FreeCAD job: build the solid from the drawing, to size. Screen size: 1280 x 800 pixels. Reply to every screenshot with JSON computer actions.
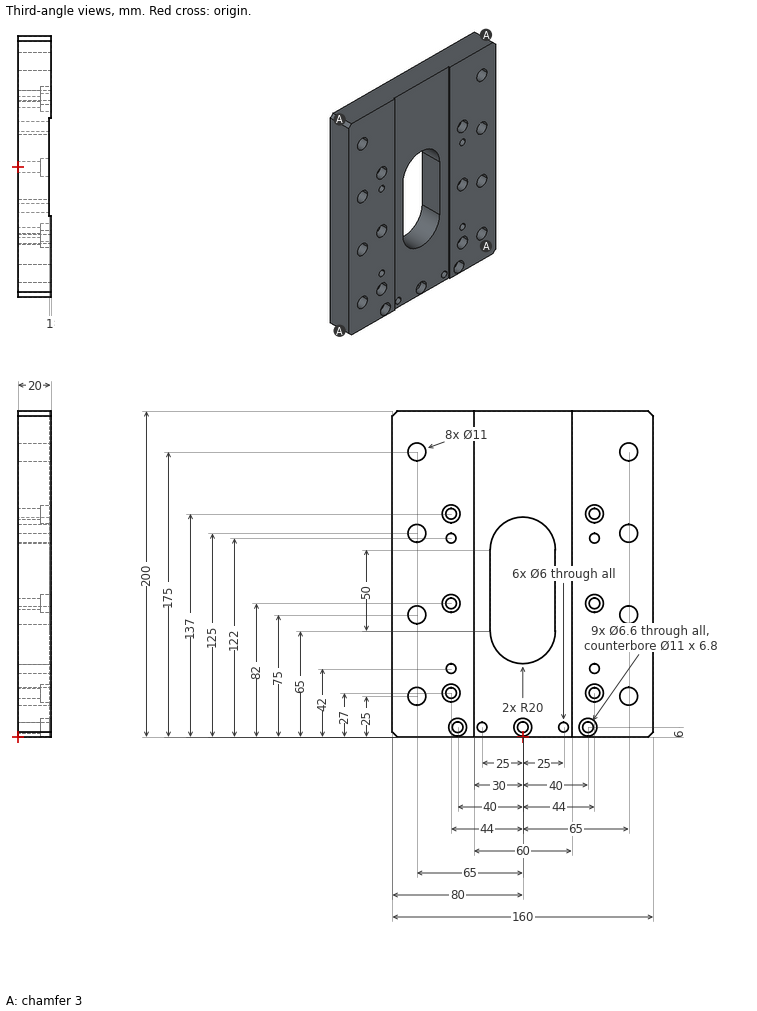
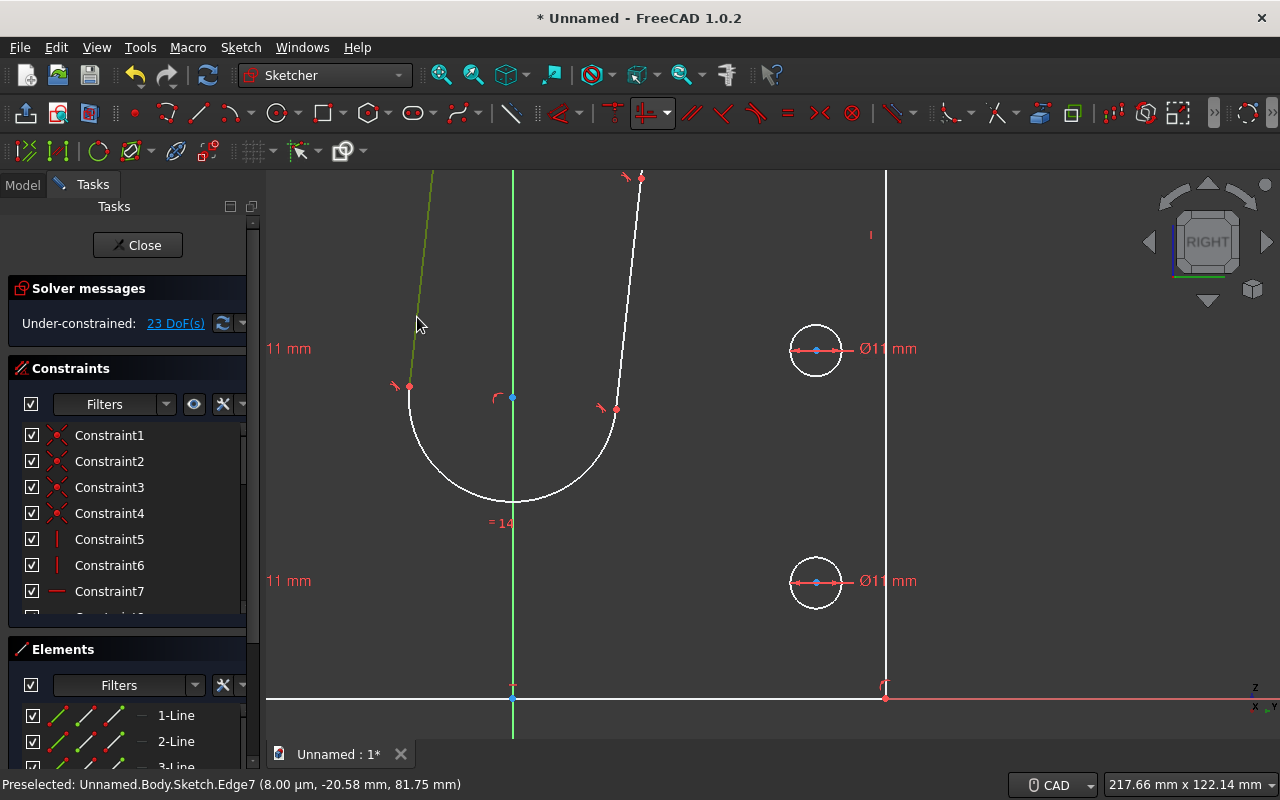
{"action": "left_click", "coordinate": [670, 114]}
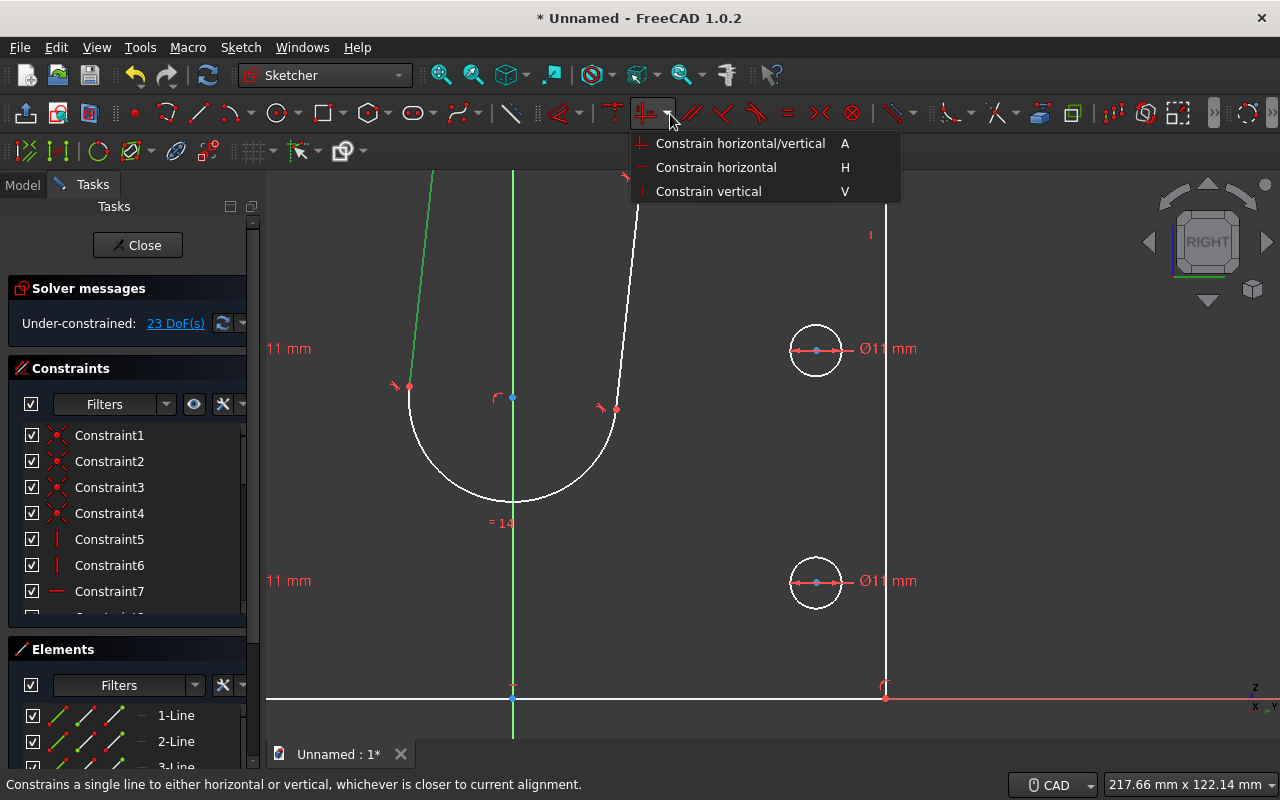
{"action": "left_click", "coordinate": [766, 191]}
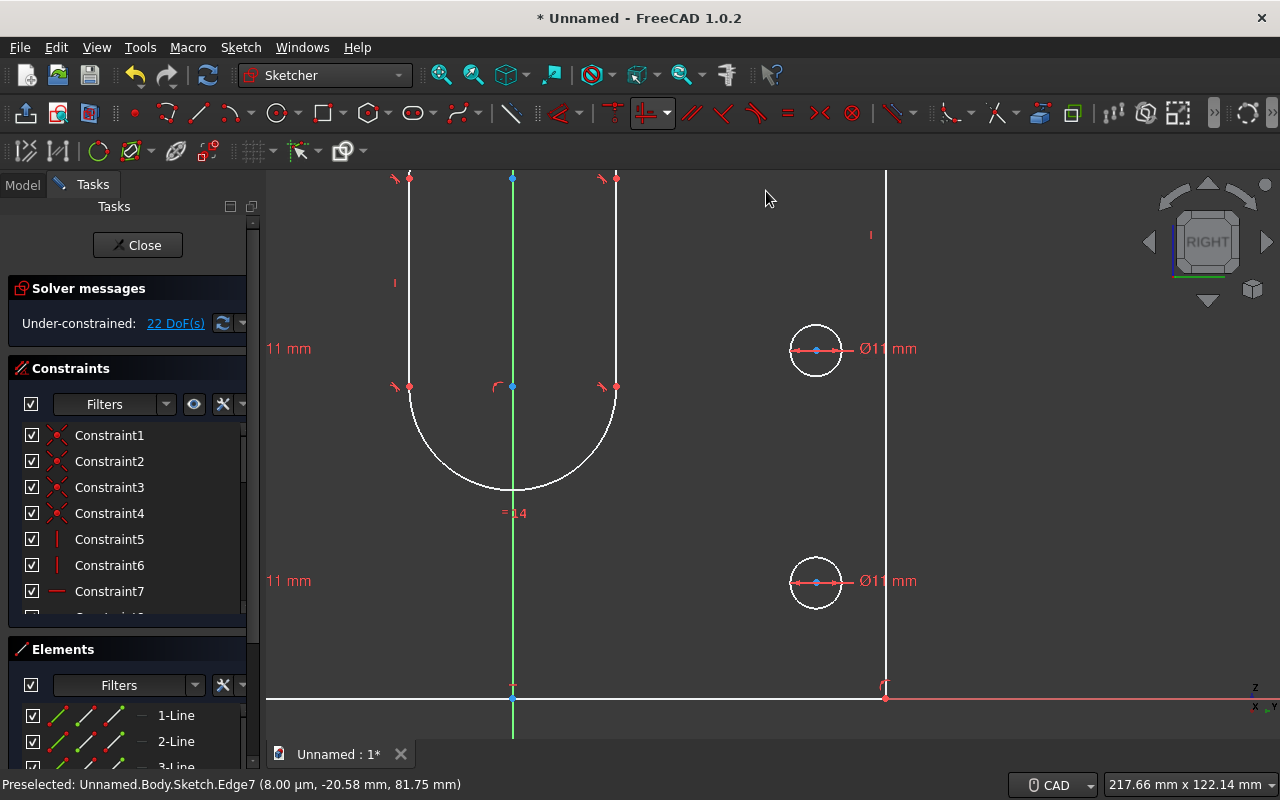
{"action": "scroll", "coordinate": [816, 583], "scroll_direction": "down", "scroll_amount": 5}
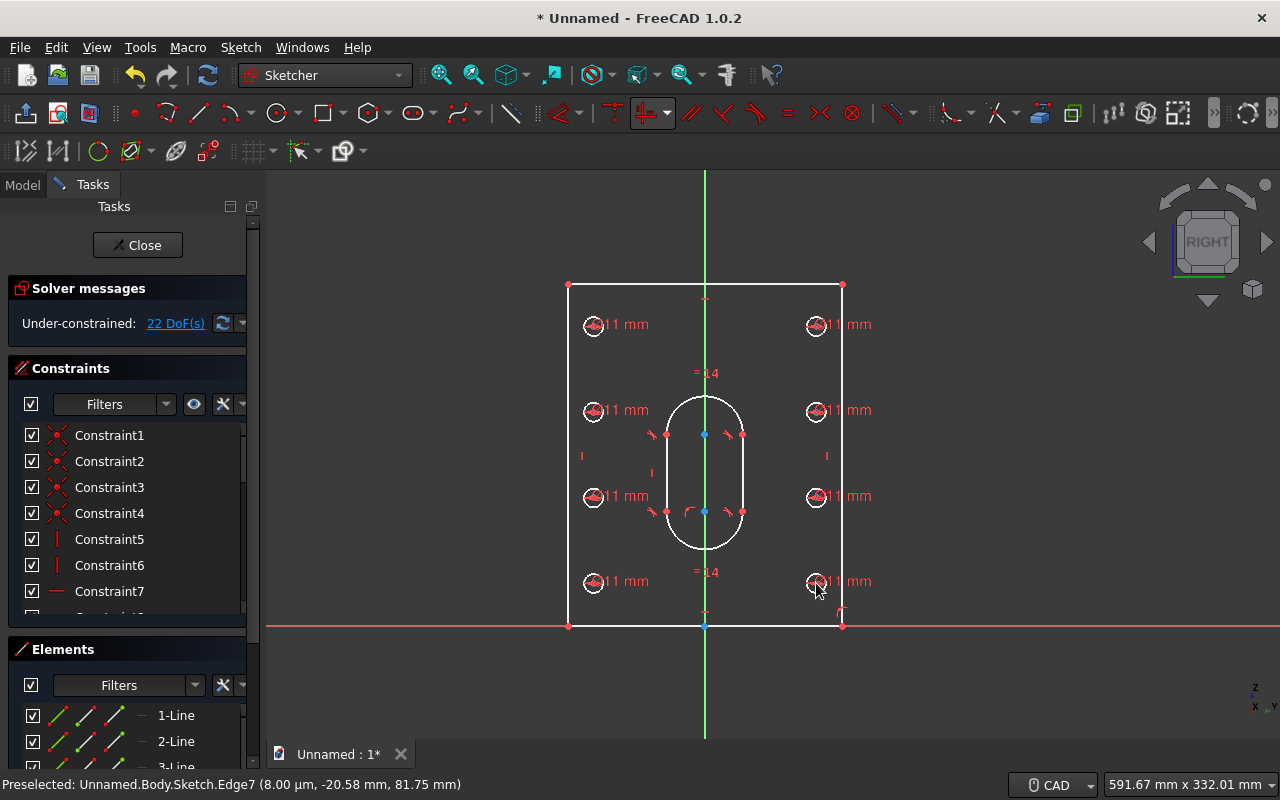
{"action": "left_click", "coordinate": [594, 327]}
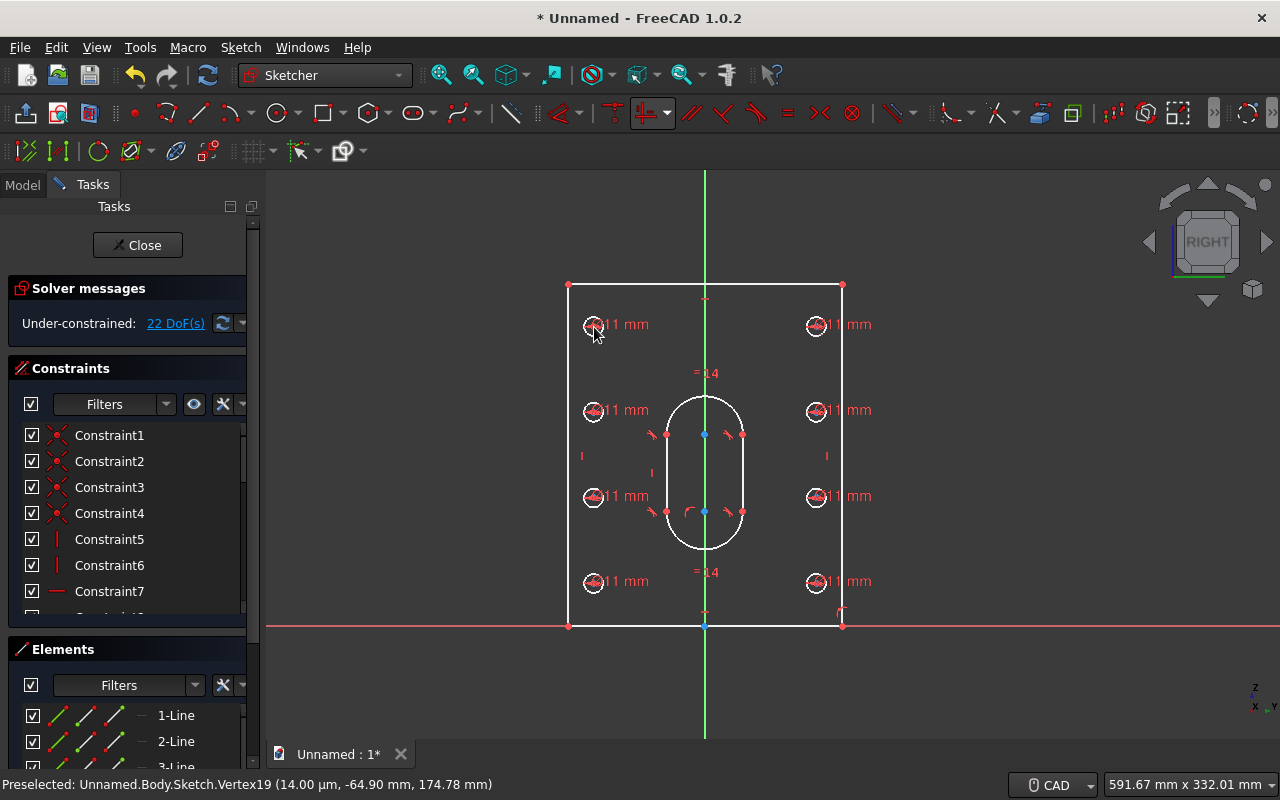
{"action": "left_click", "coordinate": [594, 412]}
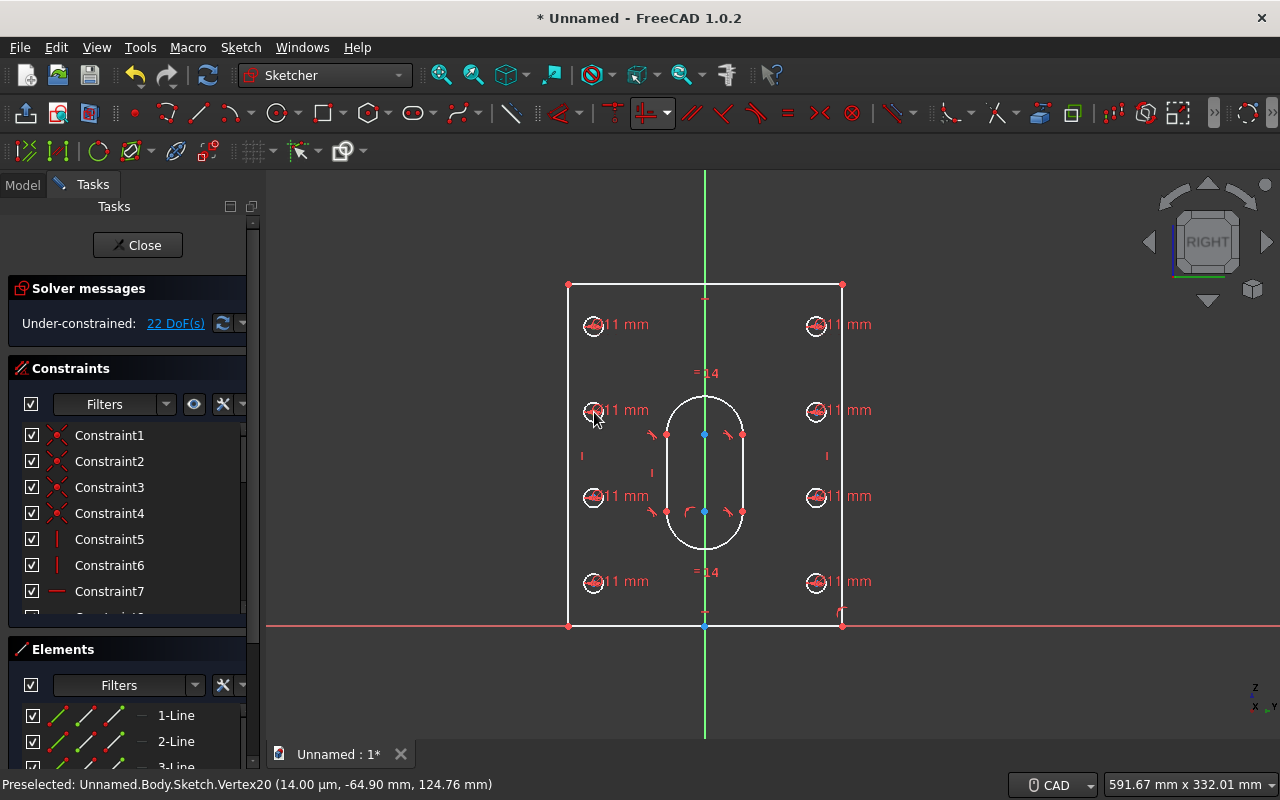
{"action": "key", "text": "v"}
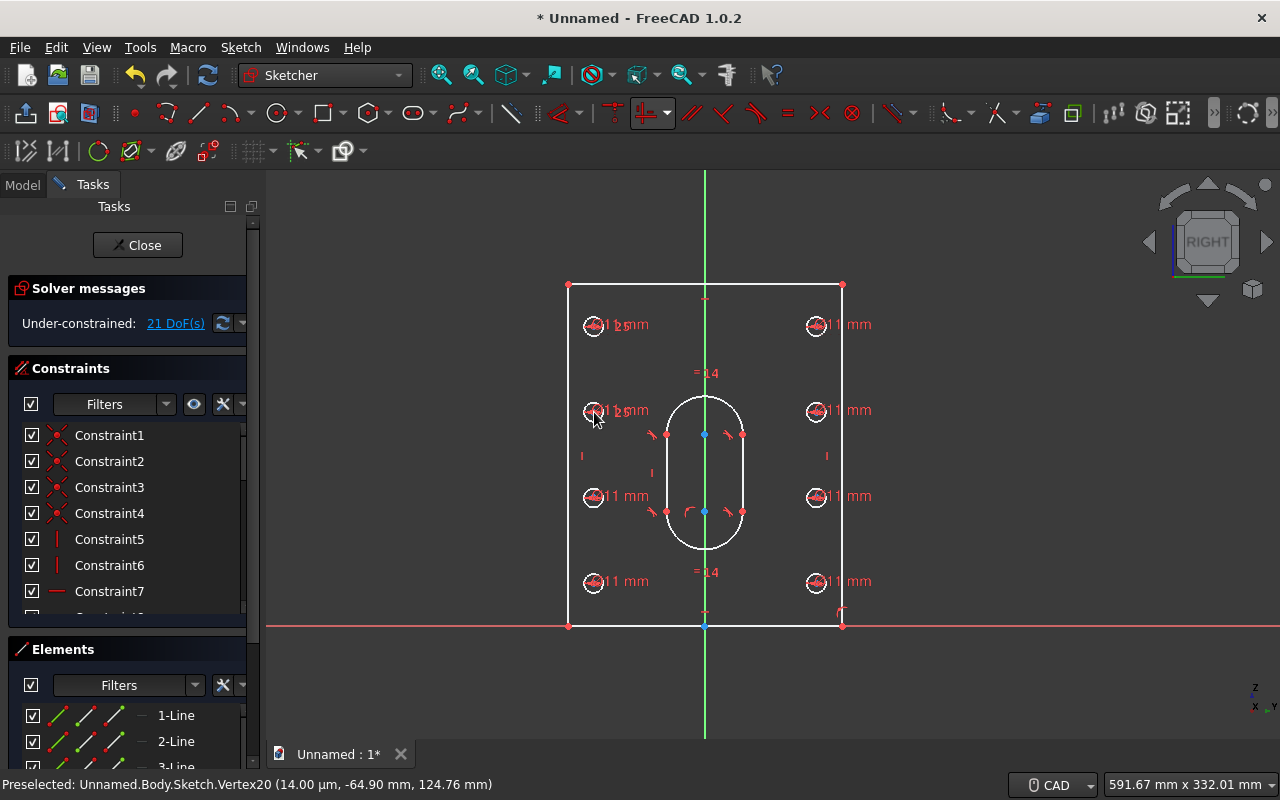
{"action": "left_click", "coordinate": [594, 412]}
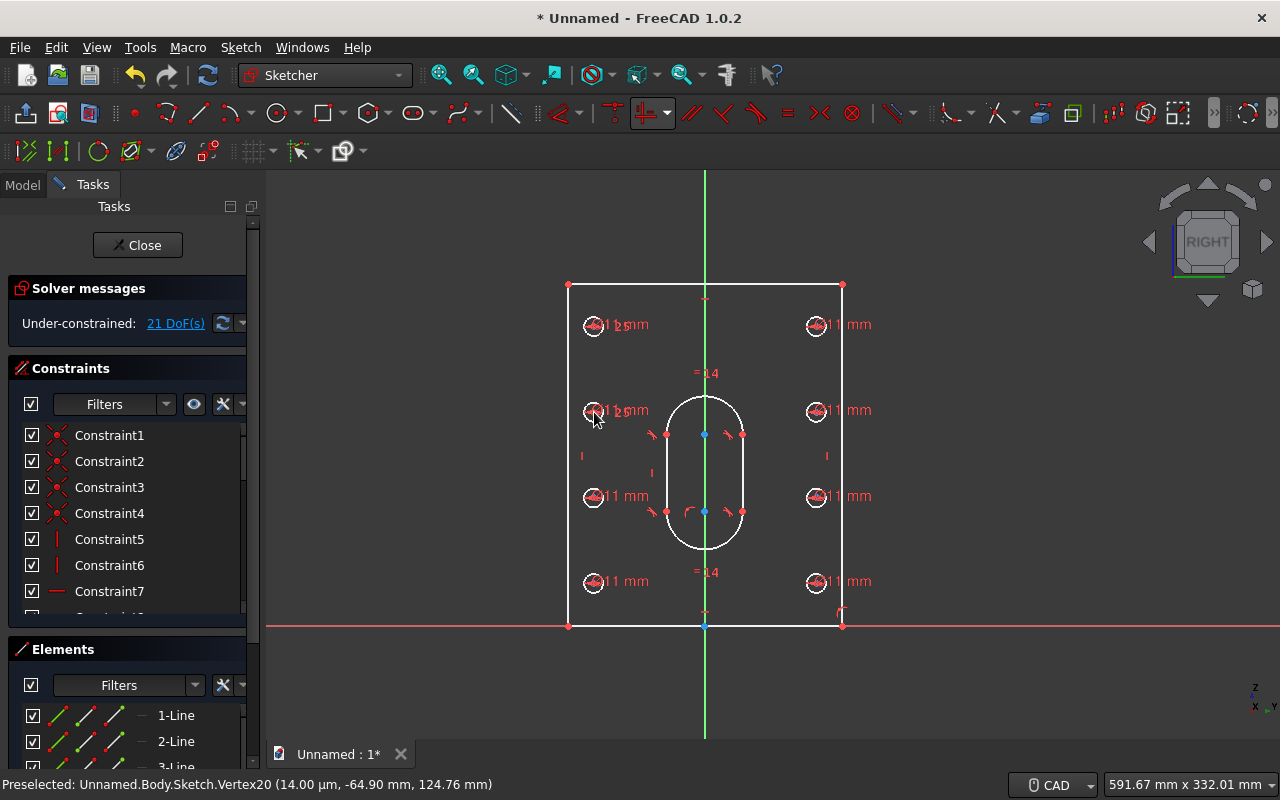
{"action": "left_click", "coordinate": [594, 498]}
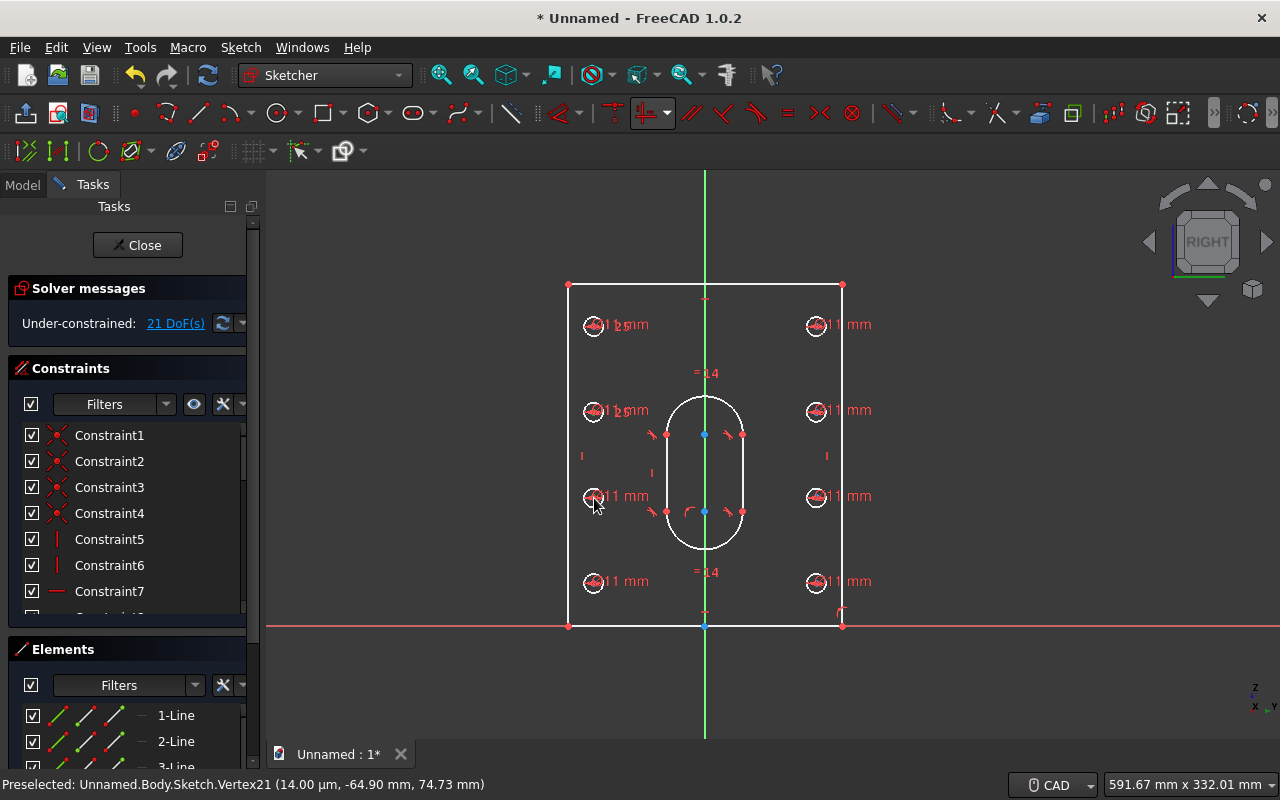
{"action": "left_click", "coordinate": [670, 114]}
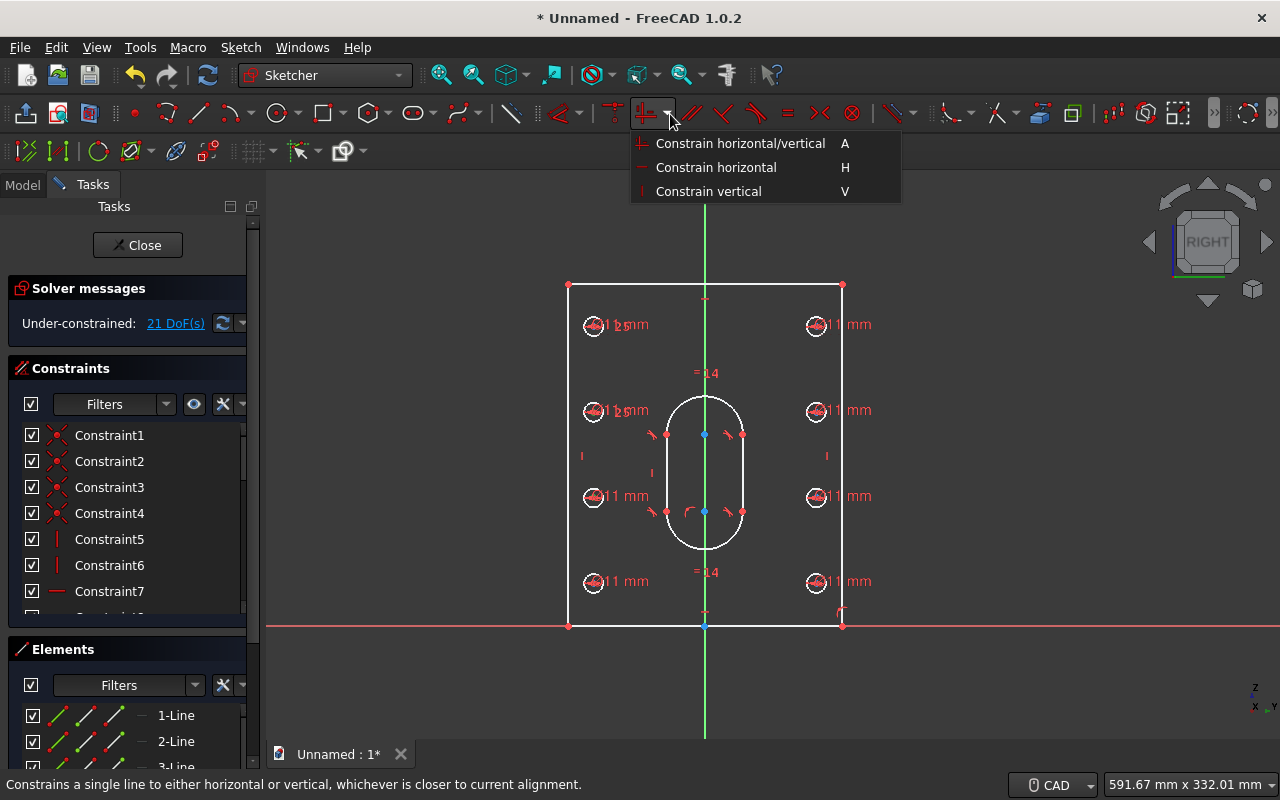
{"action": "left_click", "coordinate": [766, 191]}